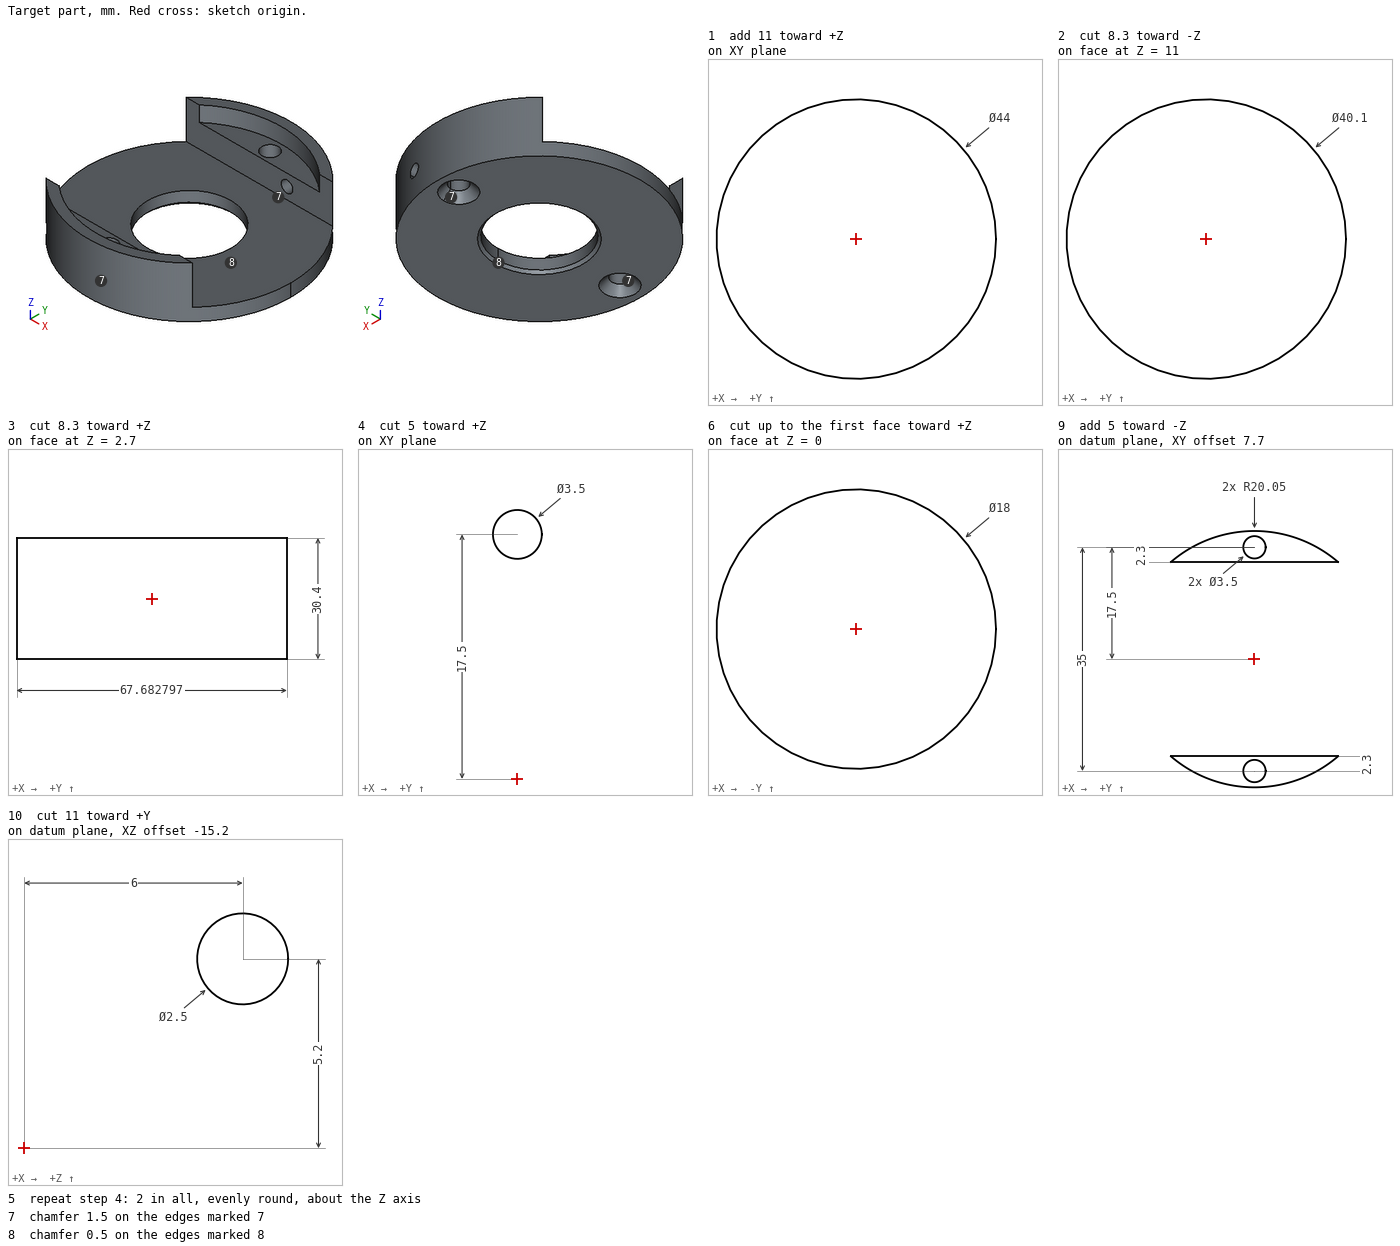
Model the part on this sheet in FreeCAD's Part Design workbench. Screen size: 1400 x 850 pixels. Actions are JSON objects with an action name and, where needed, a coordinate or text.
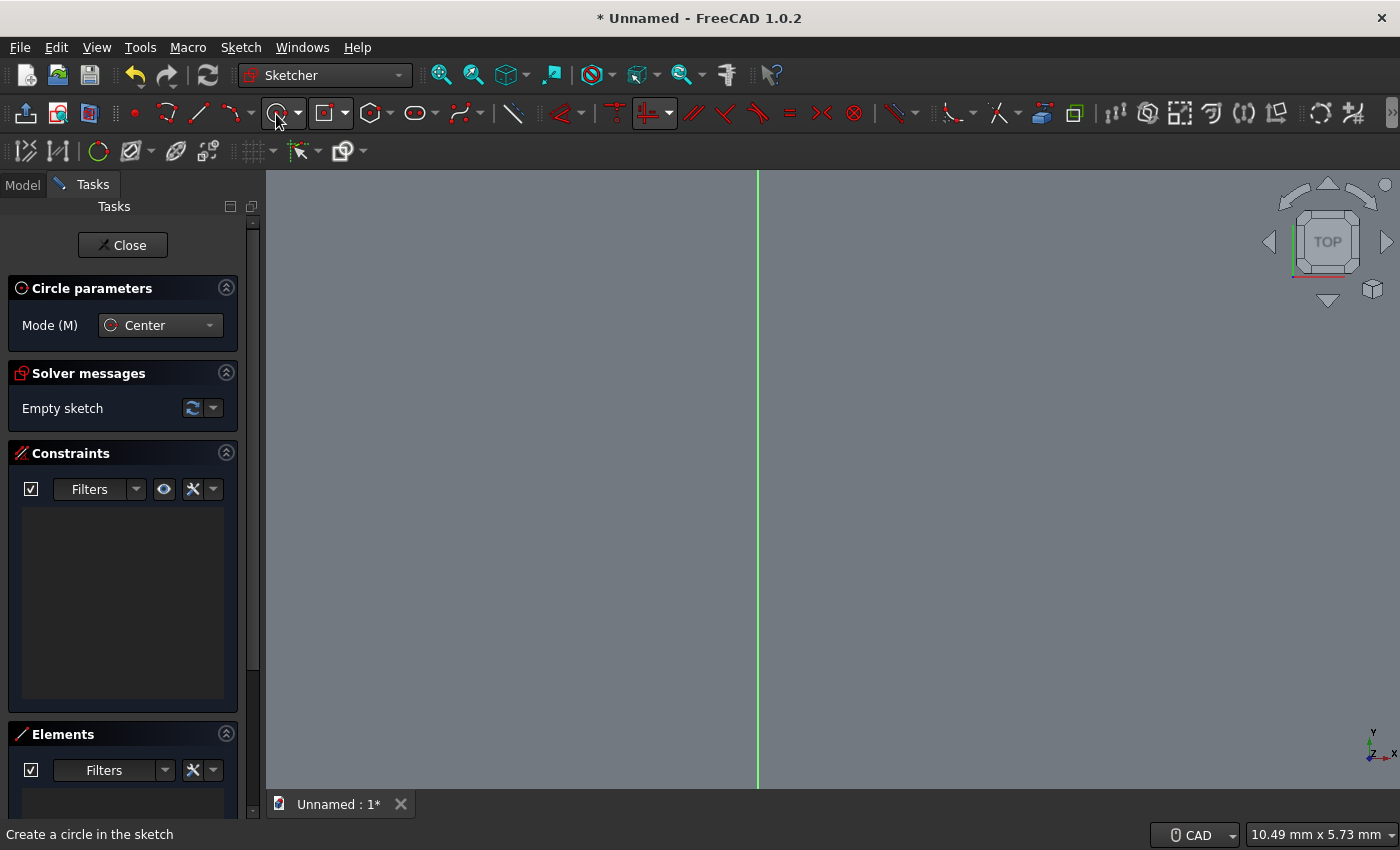
{"action": "left_click", "coordinate": [758, 476]}
{"action": "left_click", "coordinate": [891, 342]}
{"action": "key", "text": "Escape"}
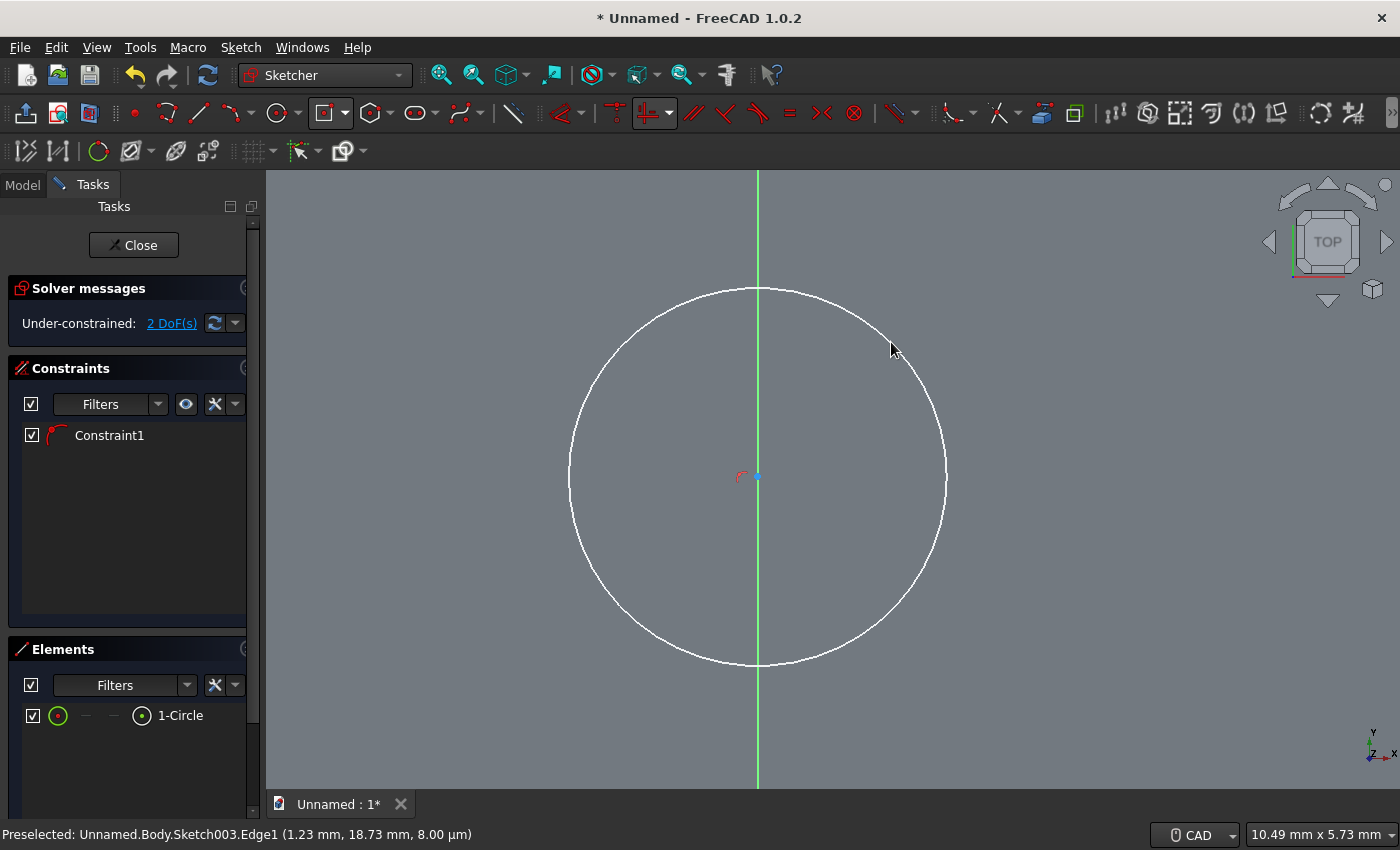
{"action": "left_click", "coordinate": [560, 114]}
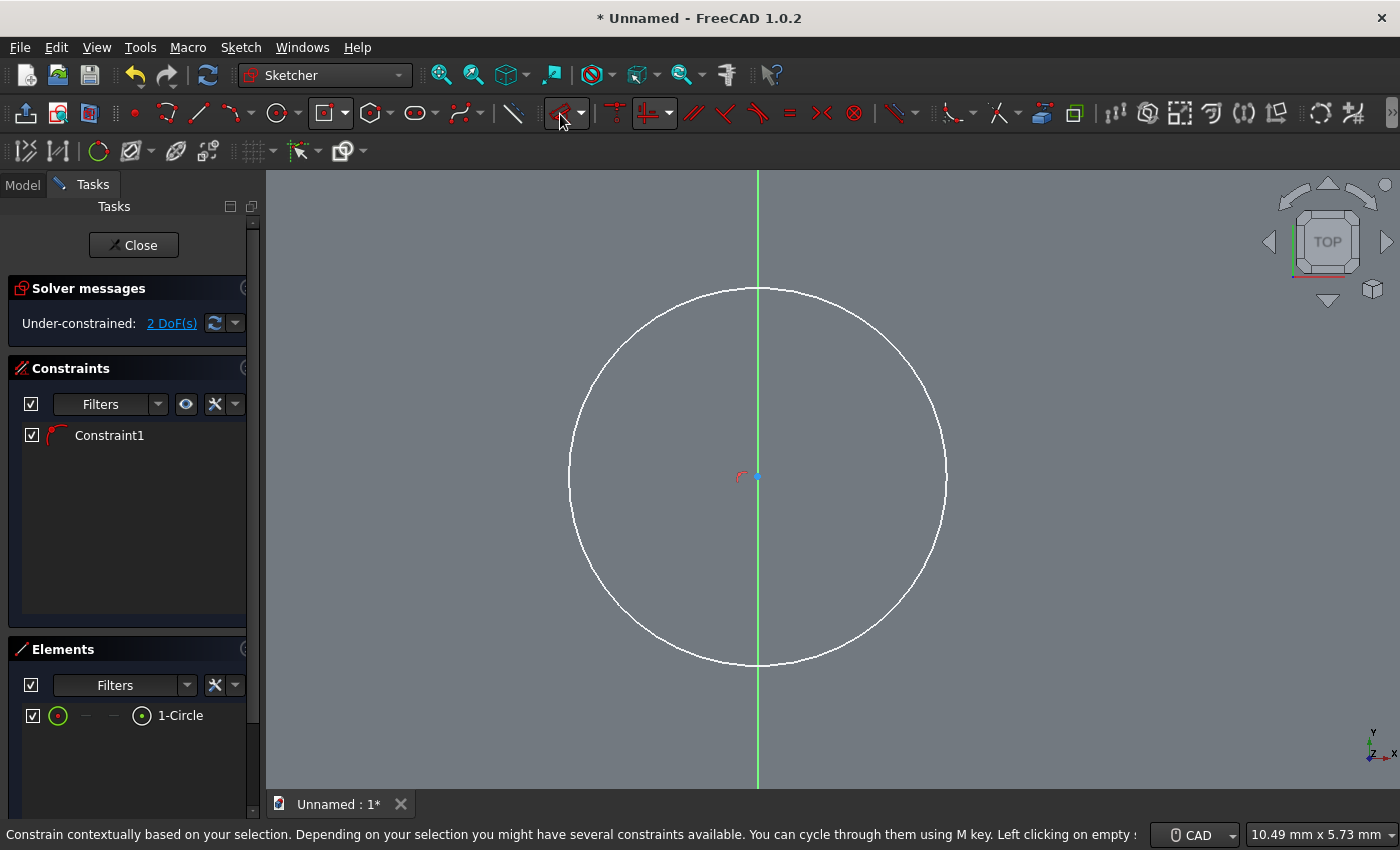
{"action": "left_click", "coordinate": [891, 343]}
{"action": "left_click", "coordinate": [914, 320]}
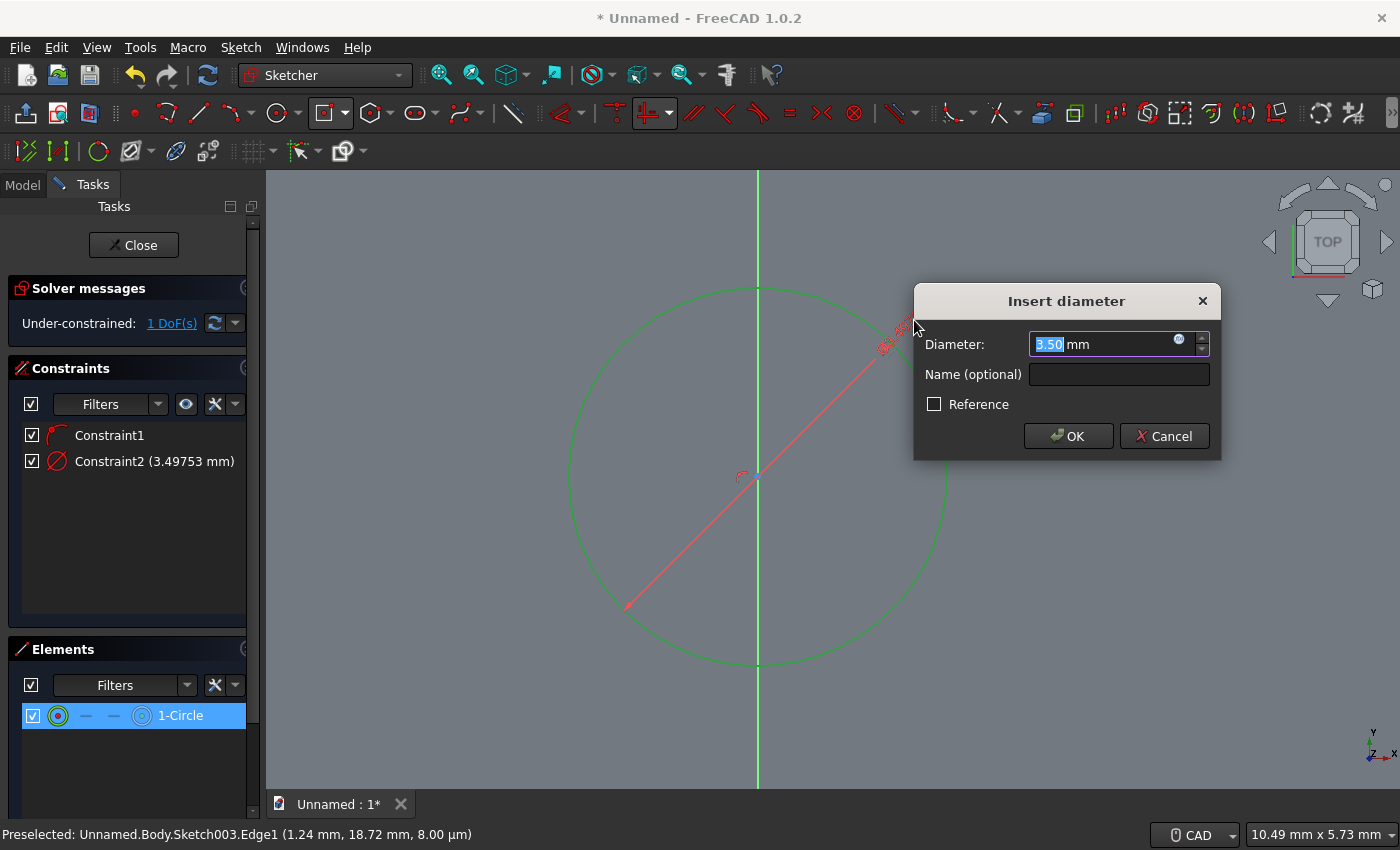
{"action": "type", "text": "3.5"}
{"action": "key", "text": "Return"}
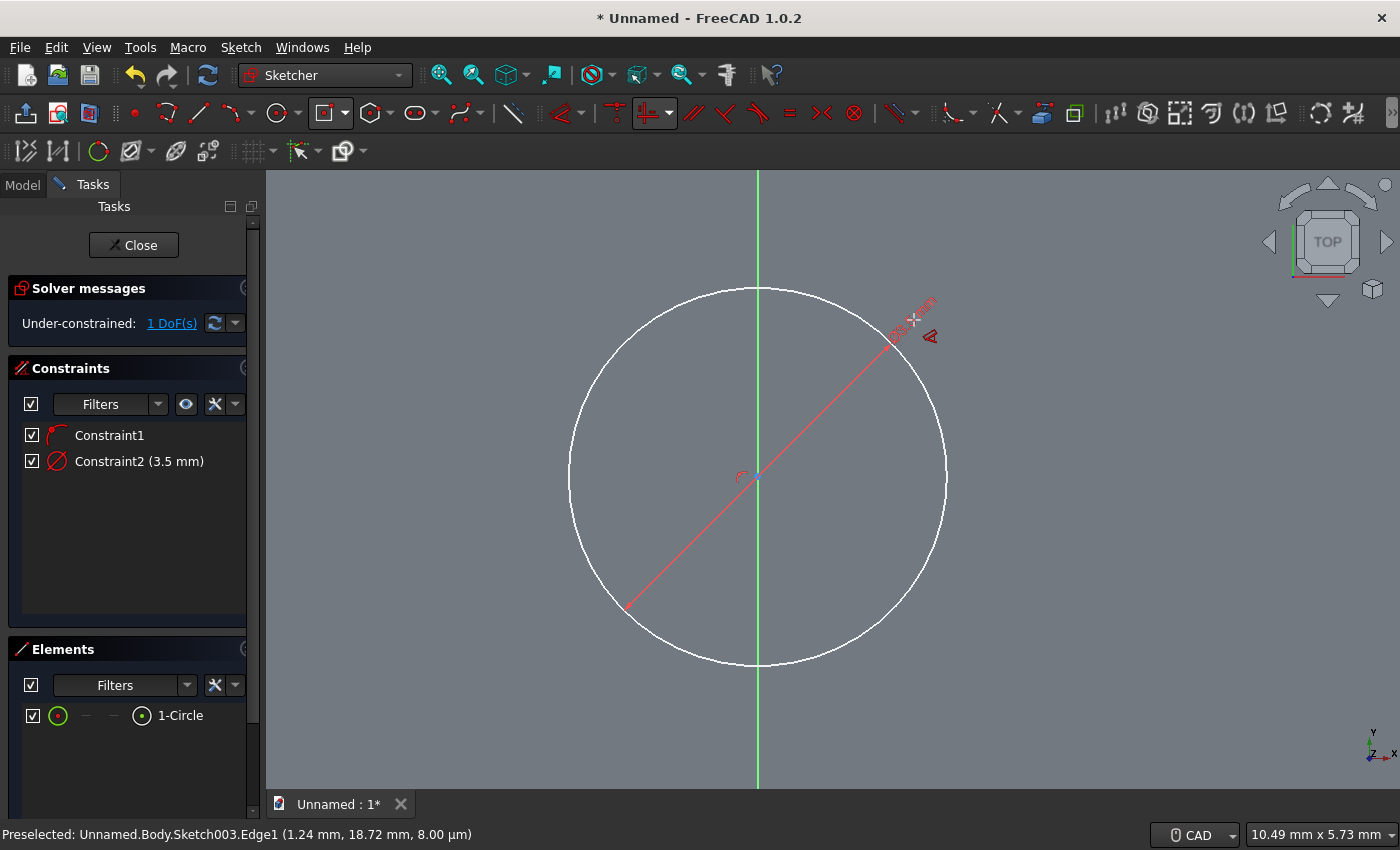
{"action": "left_click", "coordinate": [758, 477]}
{"action": "left_click", "coordinate": [792, 619]}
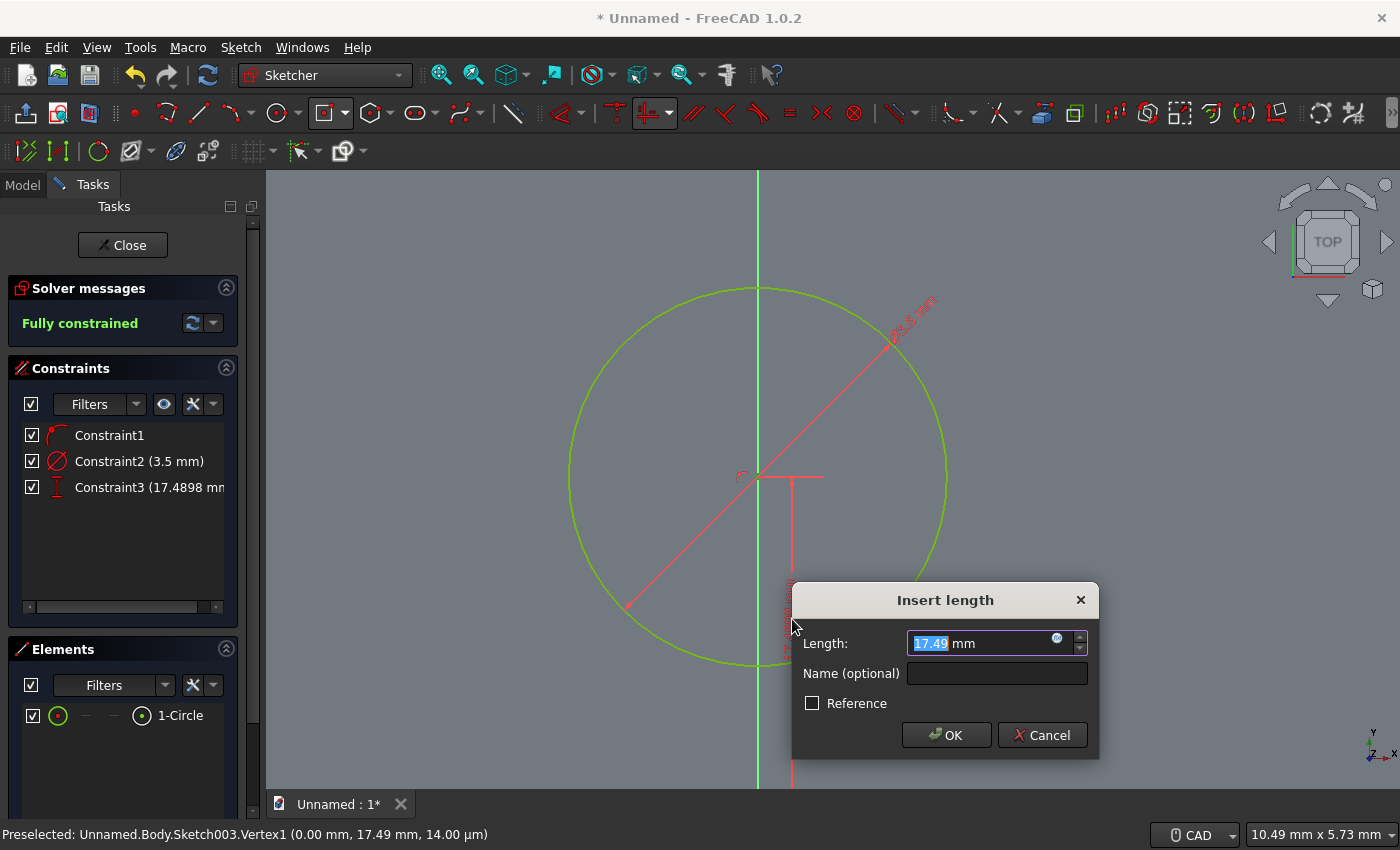
{"action": "type", "text": "17.5"}
{"action": "key", "text": "Return"}
{"action": "key", "text": "Escape"}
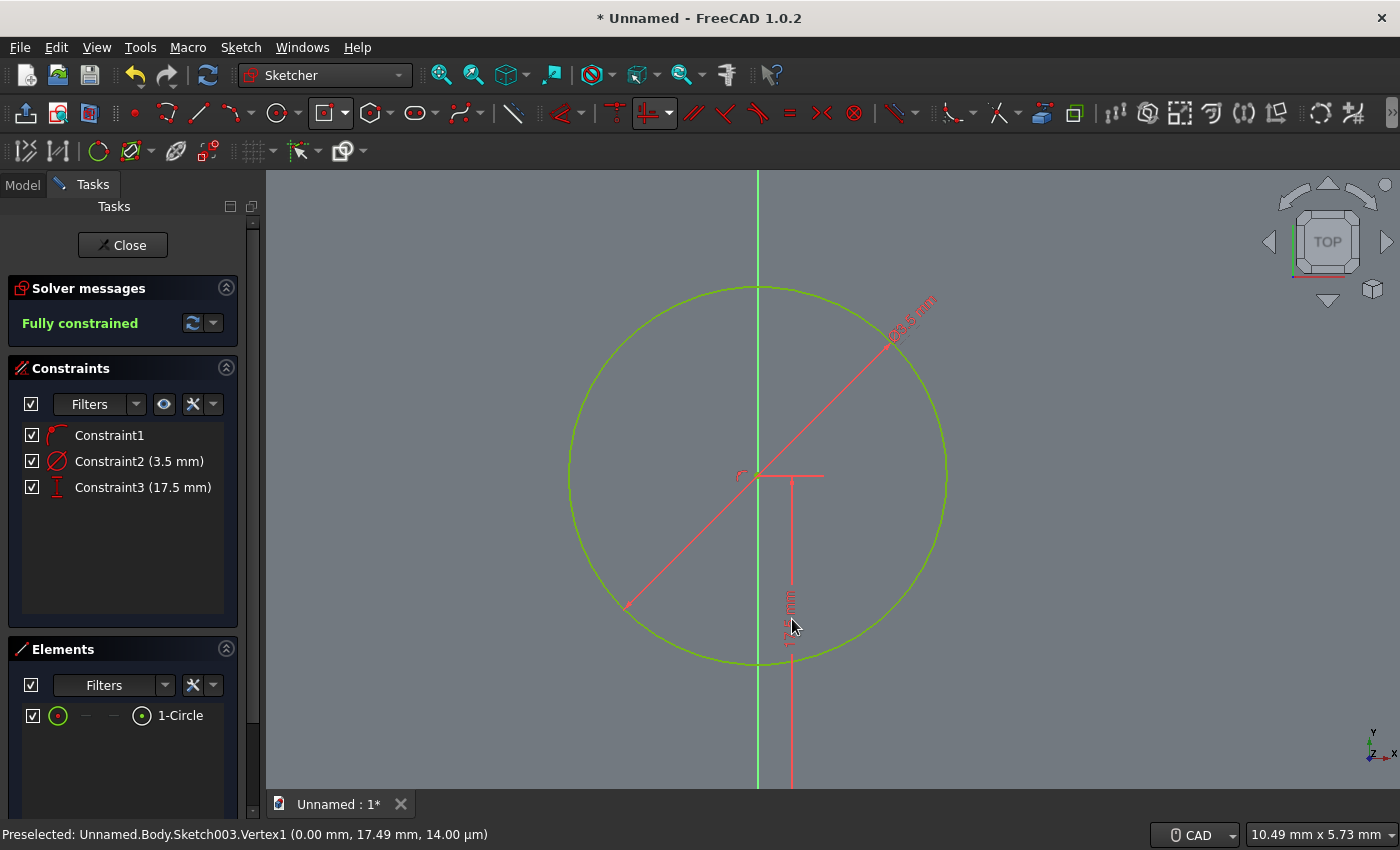
{"action": "left_click", "coordinate": [123, 245]}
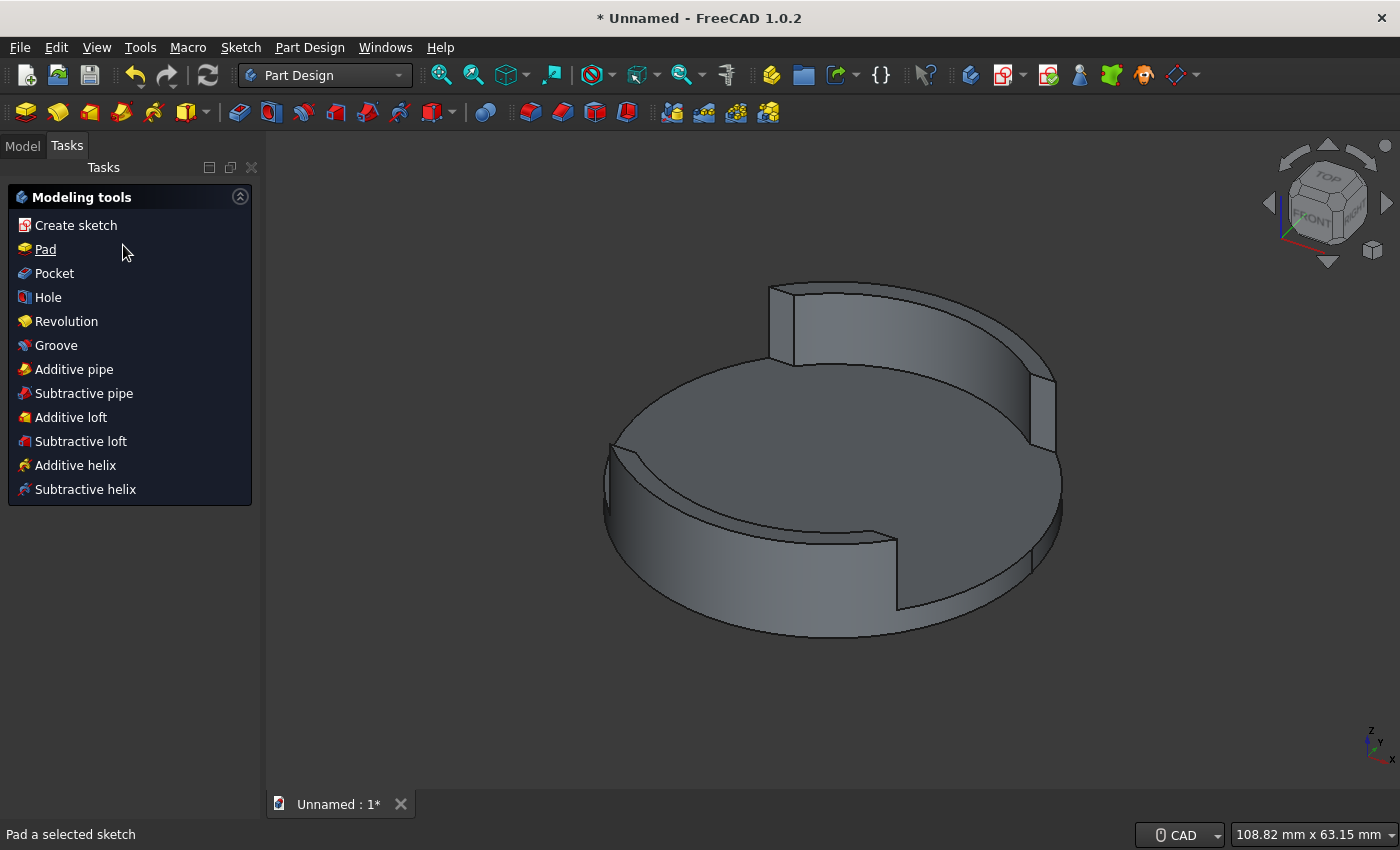
{"action": "left_click", "coordinate": [240, 112]}